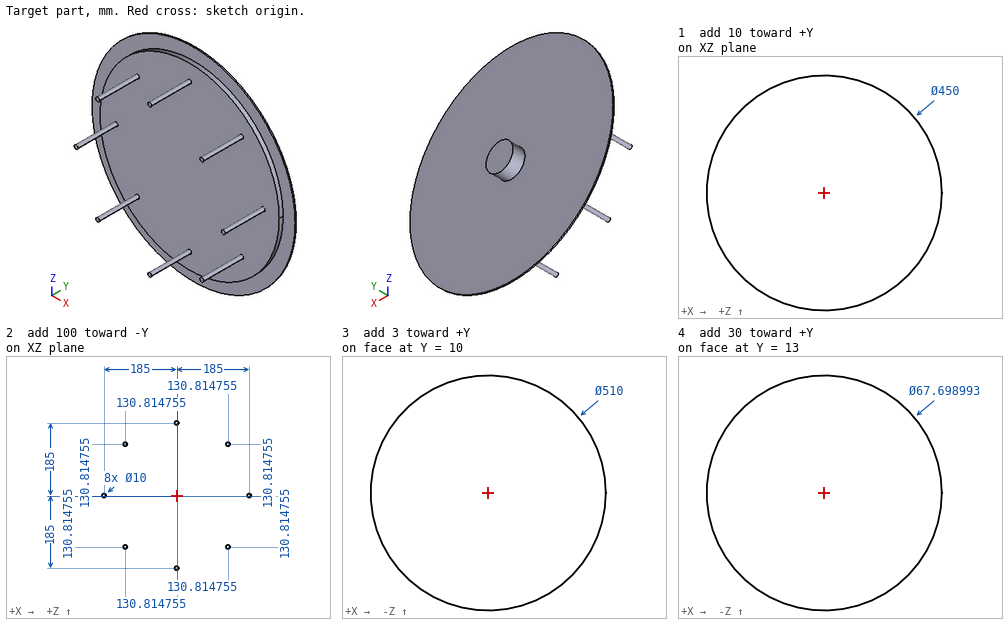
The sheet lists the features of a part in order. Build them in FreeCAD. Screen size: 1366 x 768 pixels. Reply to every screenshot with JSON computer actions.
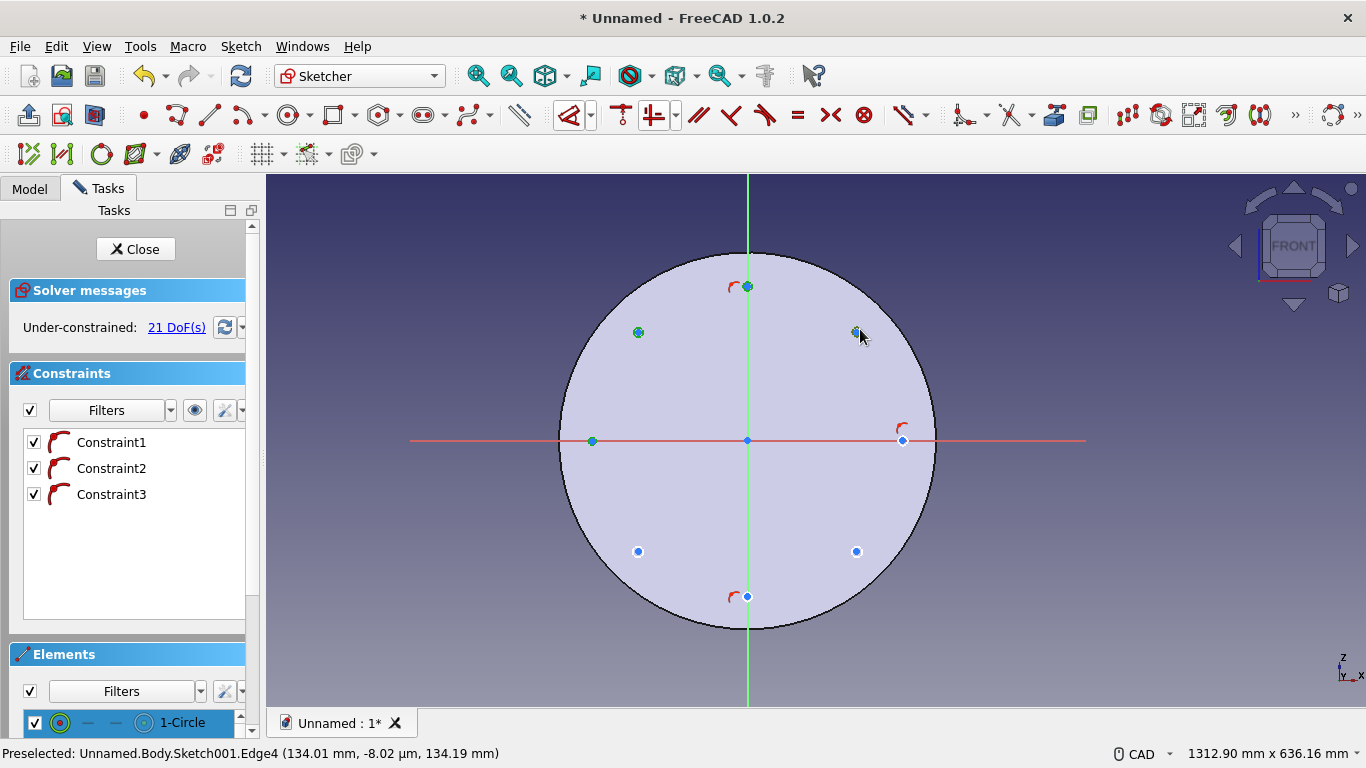
{"action": "scroll", "coordinate": [906, 438], "scroll_direction": "up", "scroll_amount": 8}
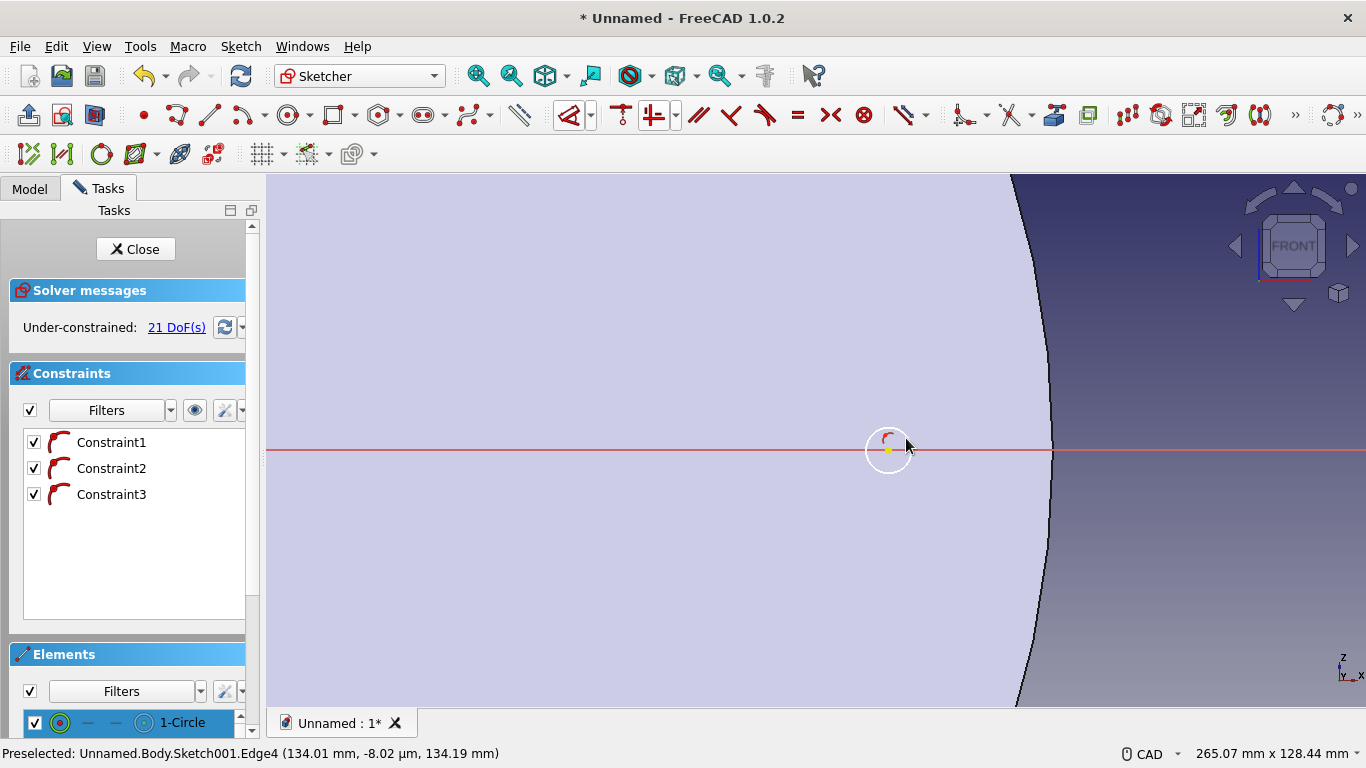
{"action": "left_click", "coordinate": [905, 434]}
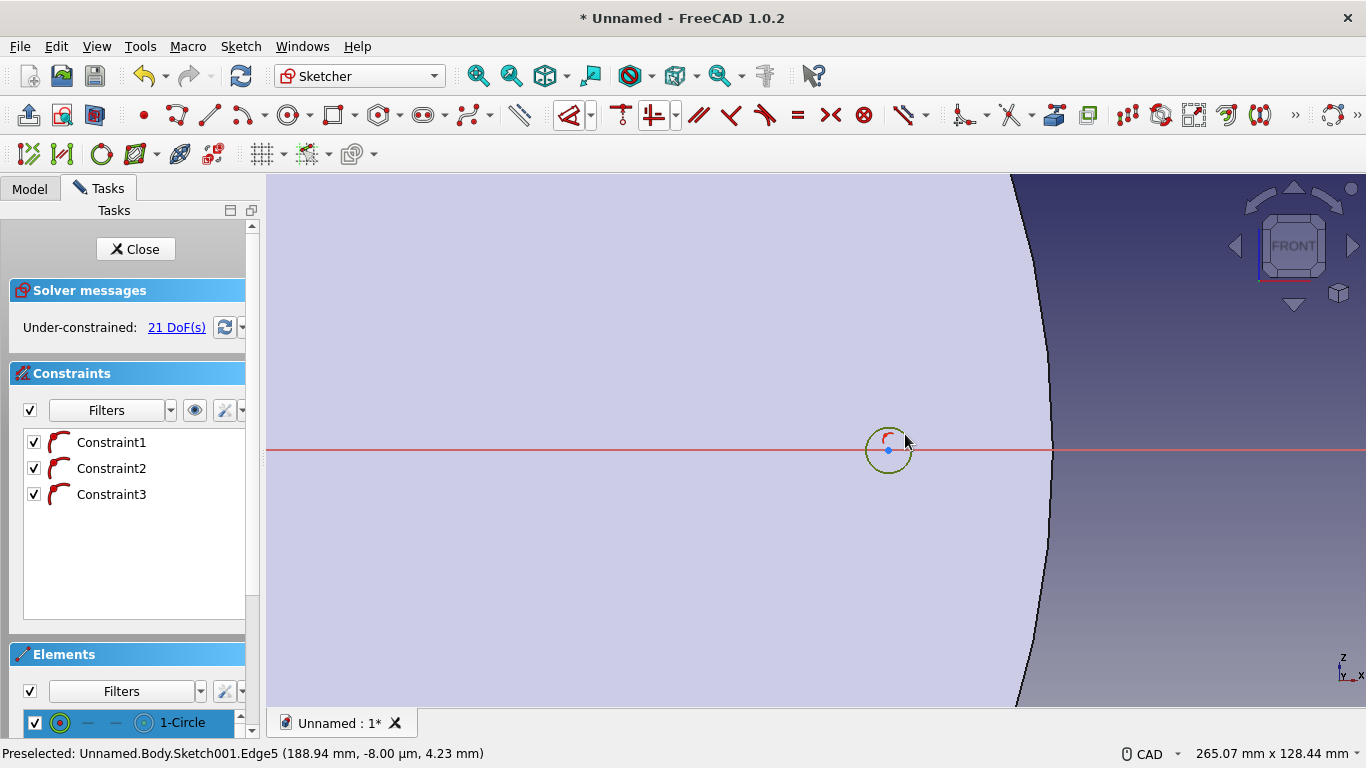
{"action": "scroll", "coordinate": [906, 438], "scroll_direction": "down", "scroll_amount": 8}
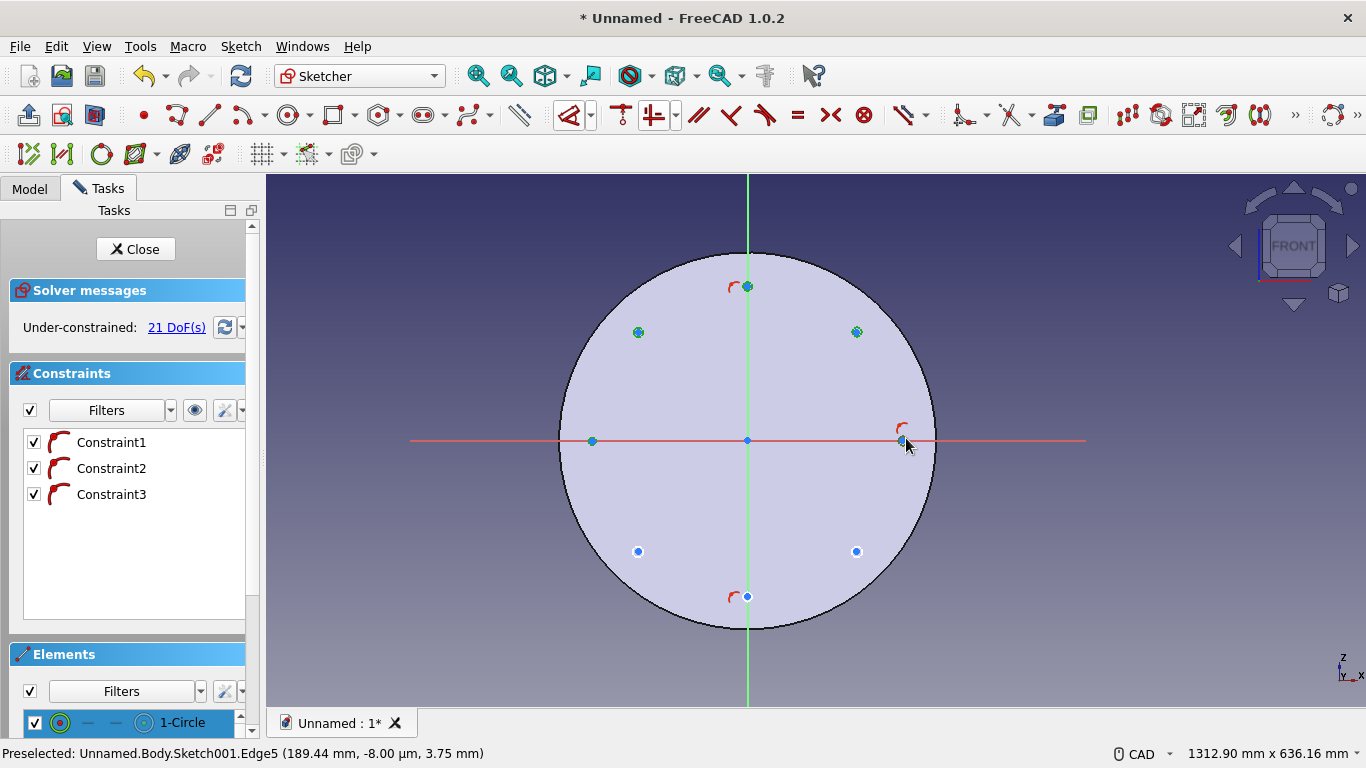
{"action": "scroll", "coordinate": [861, 548], "scroll_direction": "up", "scroll_amount": 5}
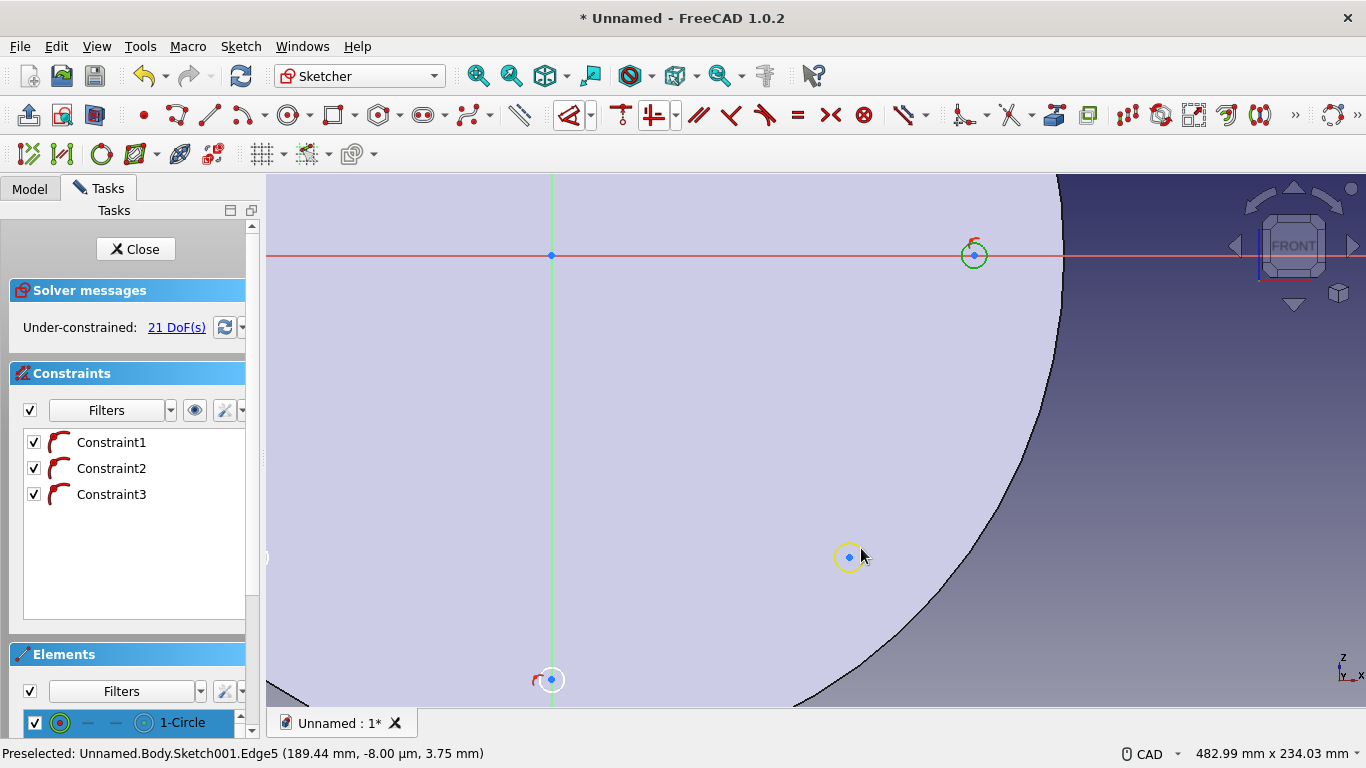
{"action": "left_click", "coordinate": [859, 548]}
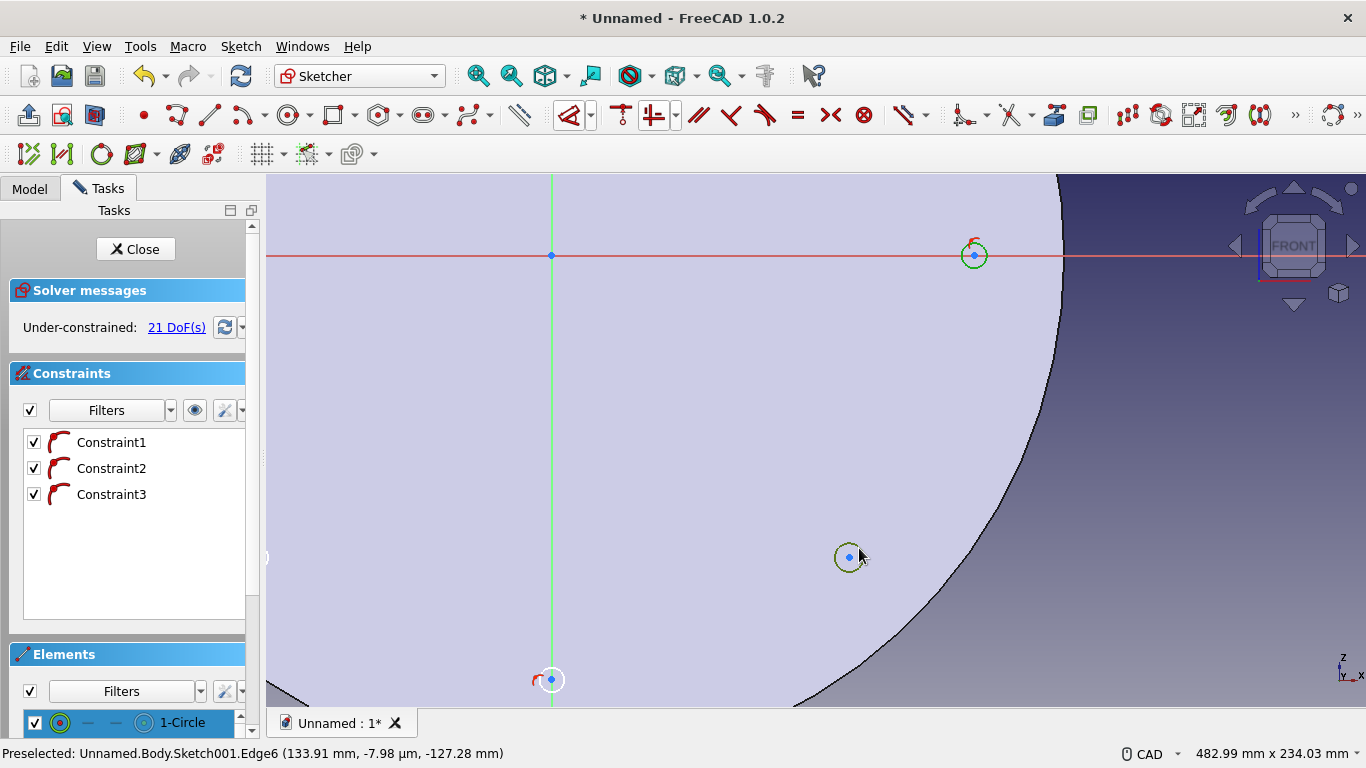
{"action": "left_click", "coordinate": [552, 668]}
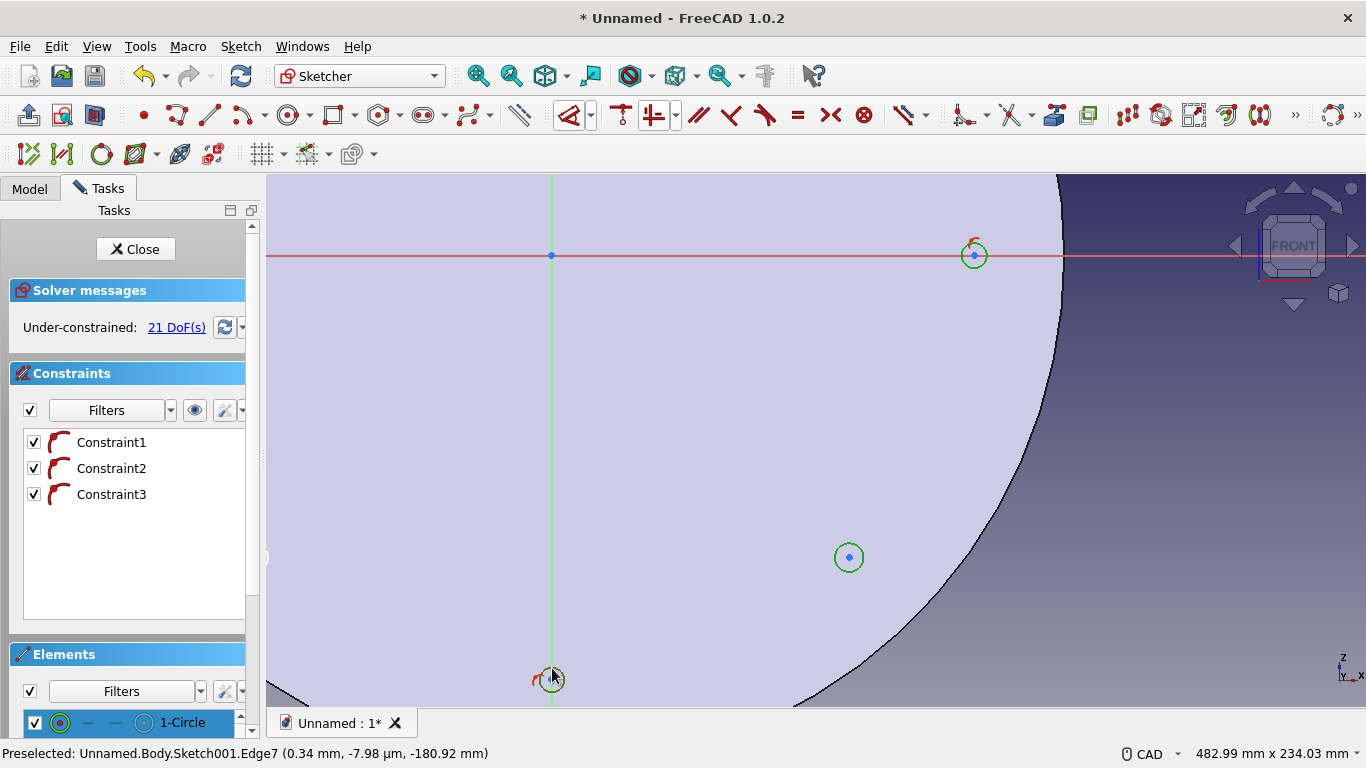
{"action": "scroll", "coordinate": [861, 548], "scroll_direction": "down", "scroll_amount": 5}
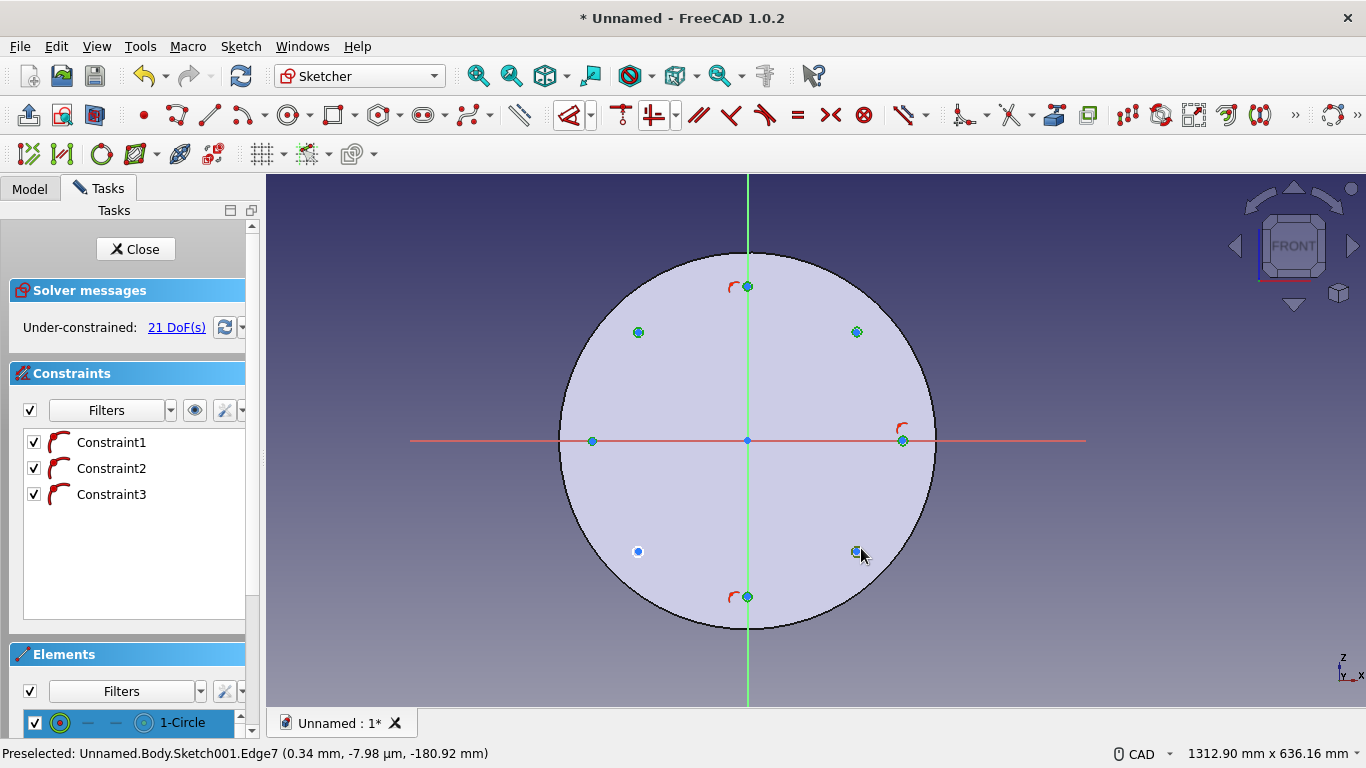
{"action": "scroll", "coordinate": [642, 548], "scroll_direction": "up", "scroll_amount": 5}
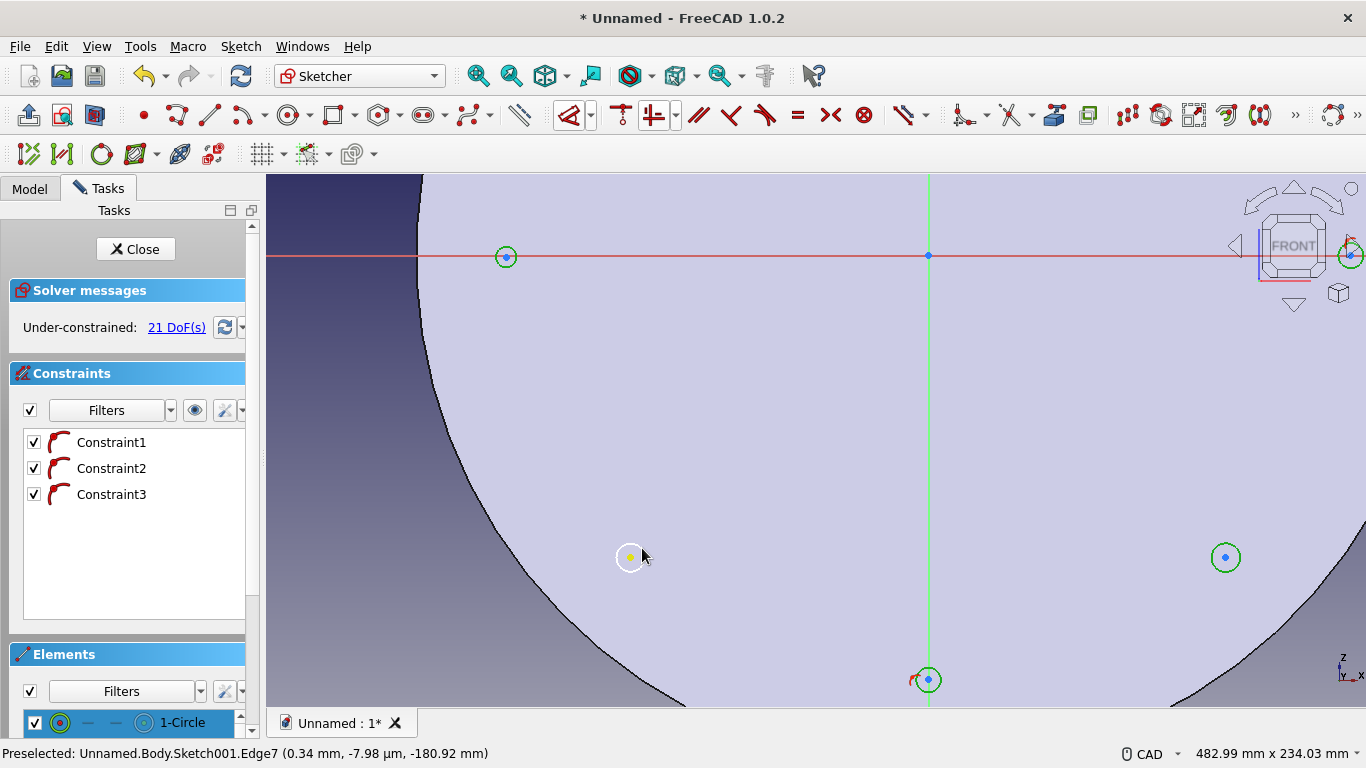
{"action": "left_click", "coordinate": [640, 548]}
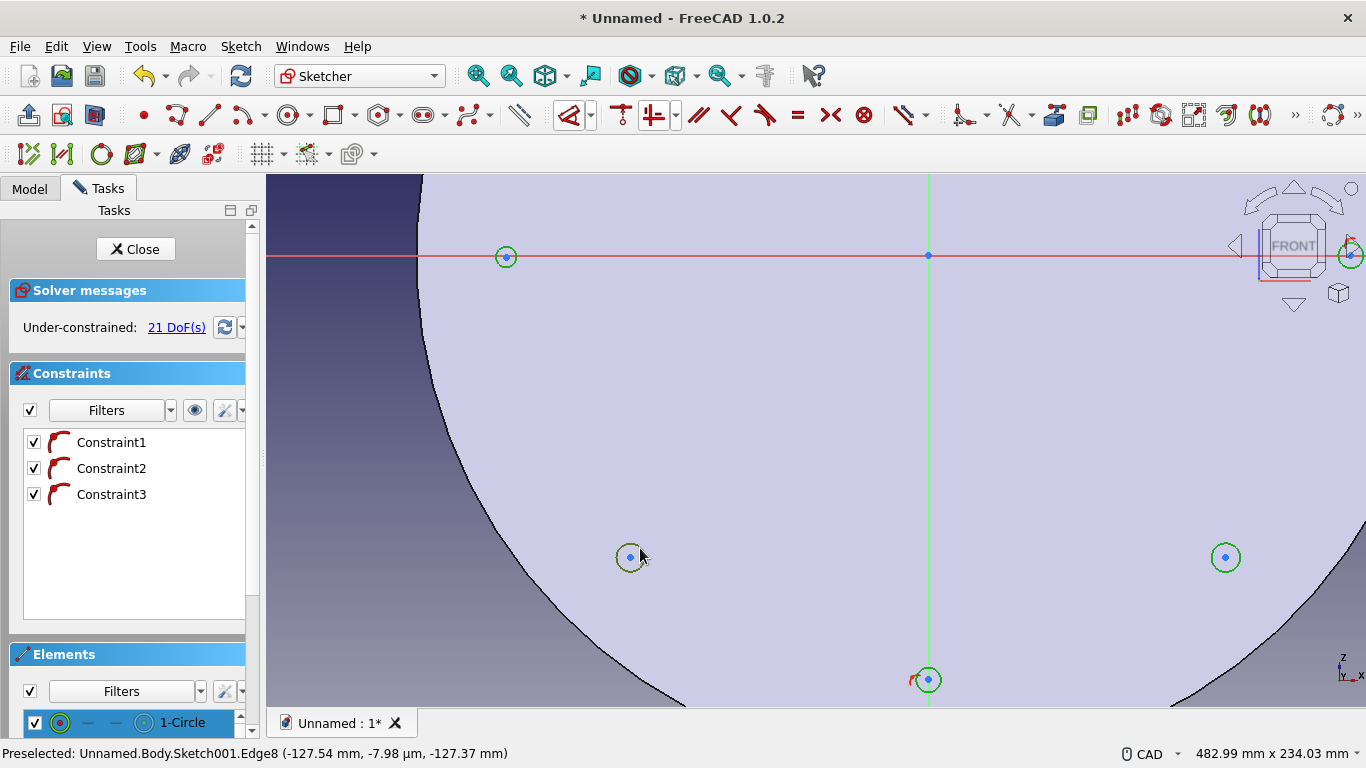
{"action": "left_click", "coordinate": [798, 116]}